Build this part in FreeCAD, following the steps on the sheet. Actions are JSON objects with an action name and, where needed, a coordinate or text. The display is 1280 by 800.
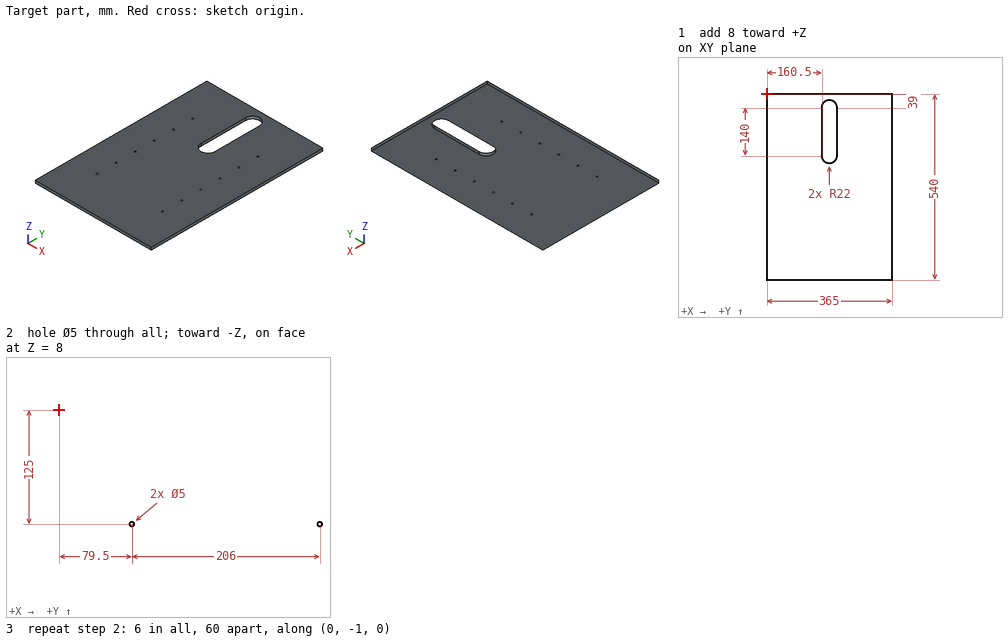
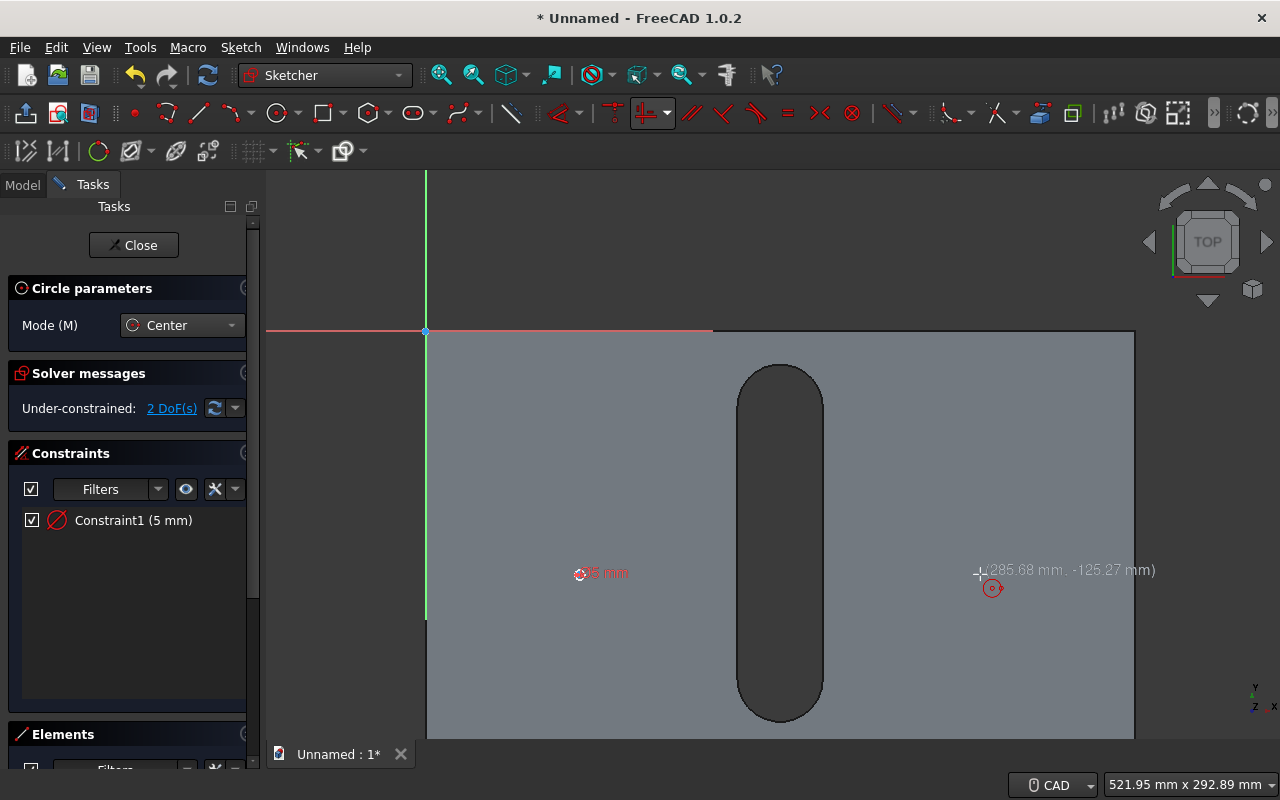
{"action": "left_click", "coordinate": [980, 574]}
{"action": "mouse_move", "coordinate": [984, 571]}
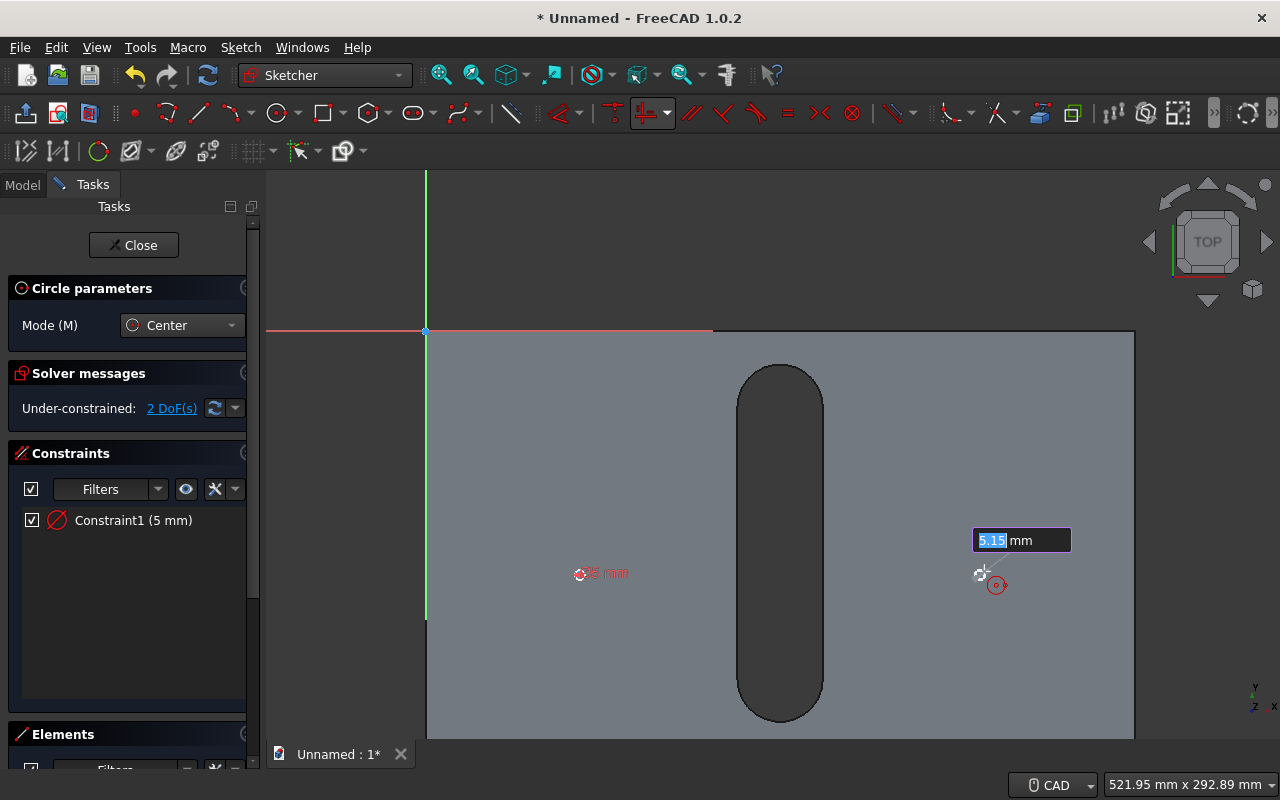
{"action": "type", "text": "5"}
{"action": "key", "text": "Return"}
{"action": "key", "text": "Escape"}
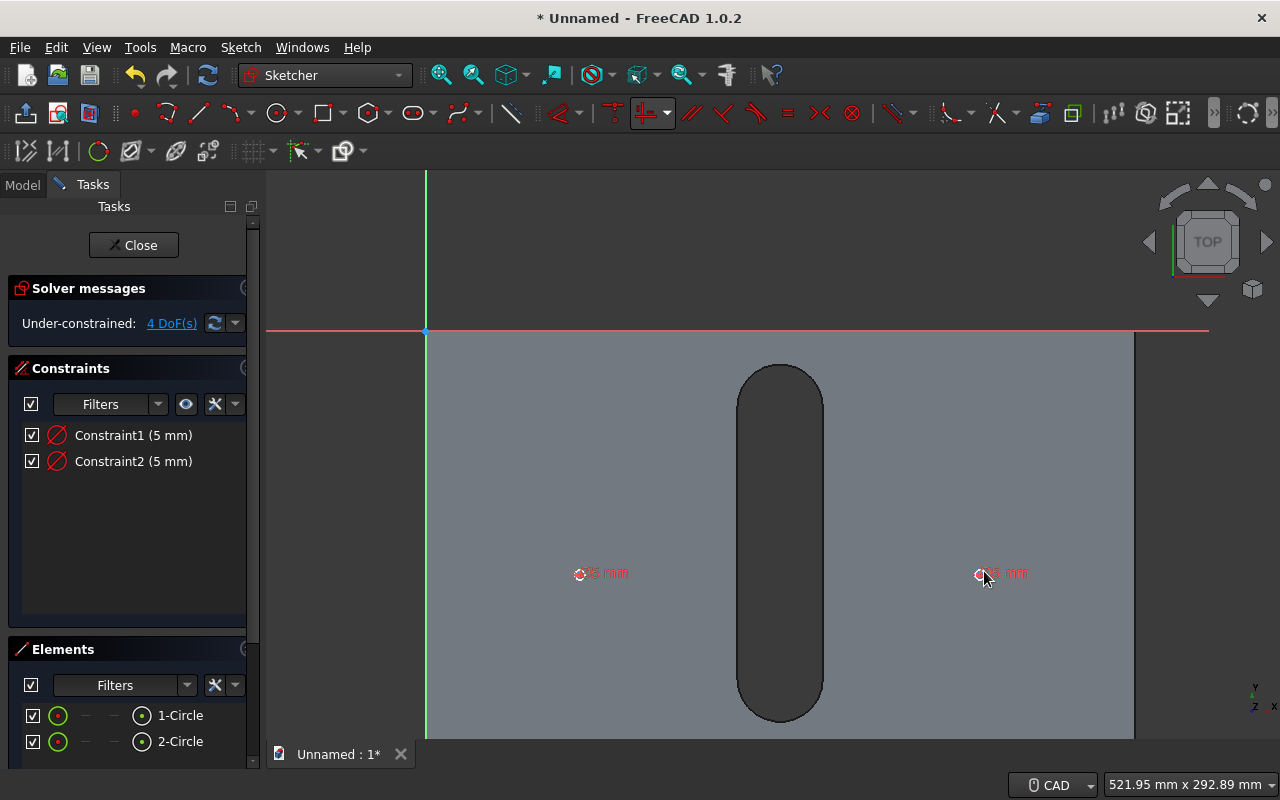
{"action": "left_click", "coordinate": [580, 575]}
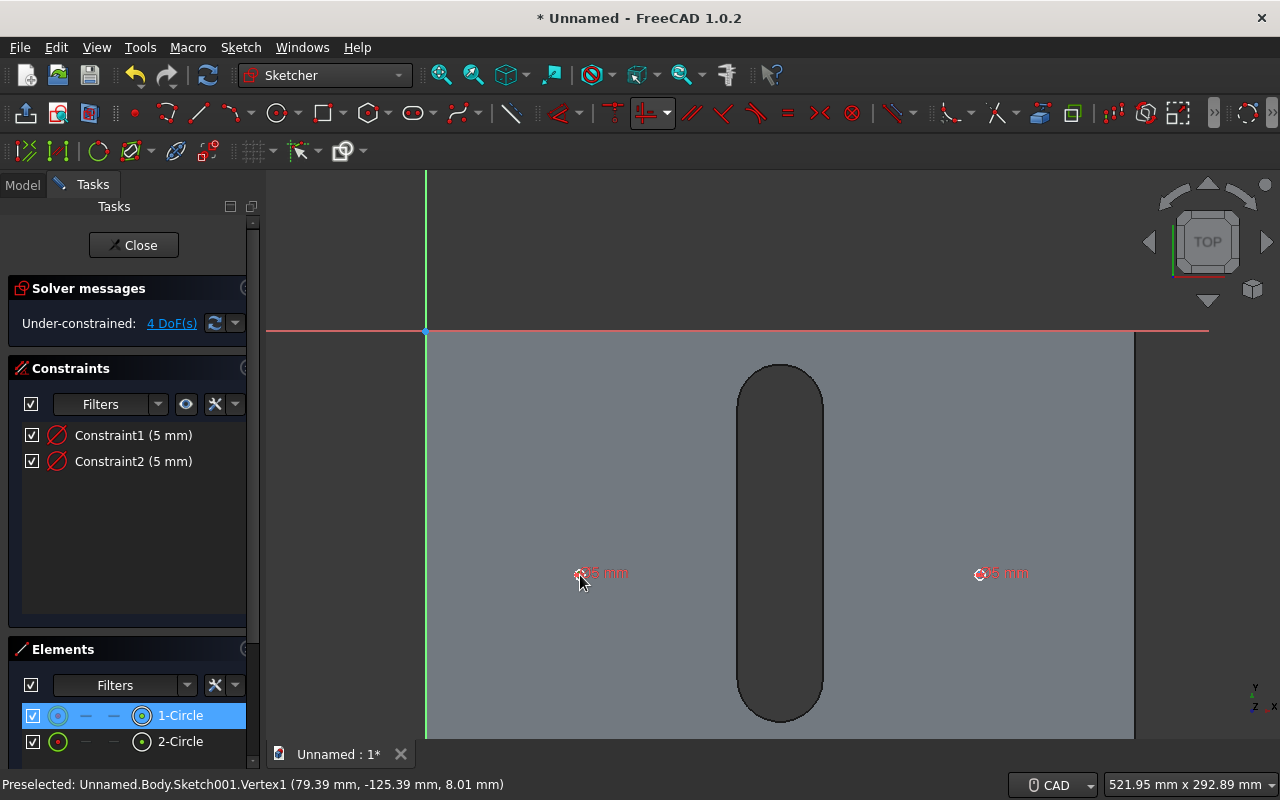
{"action": "left_click", "coordinate": [980, 575]}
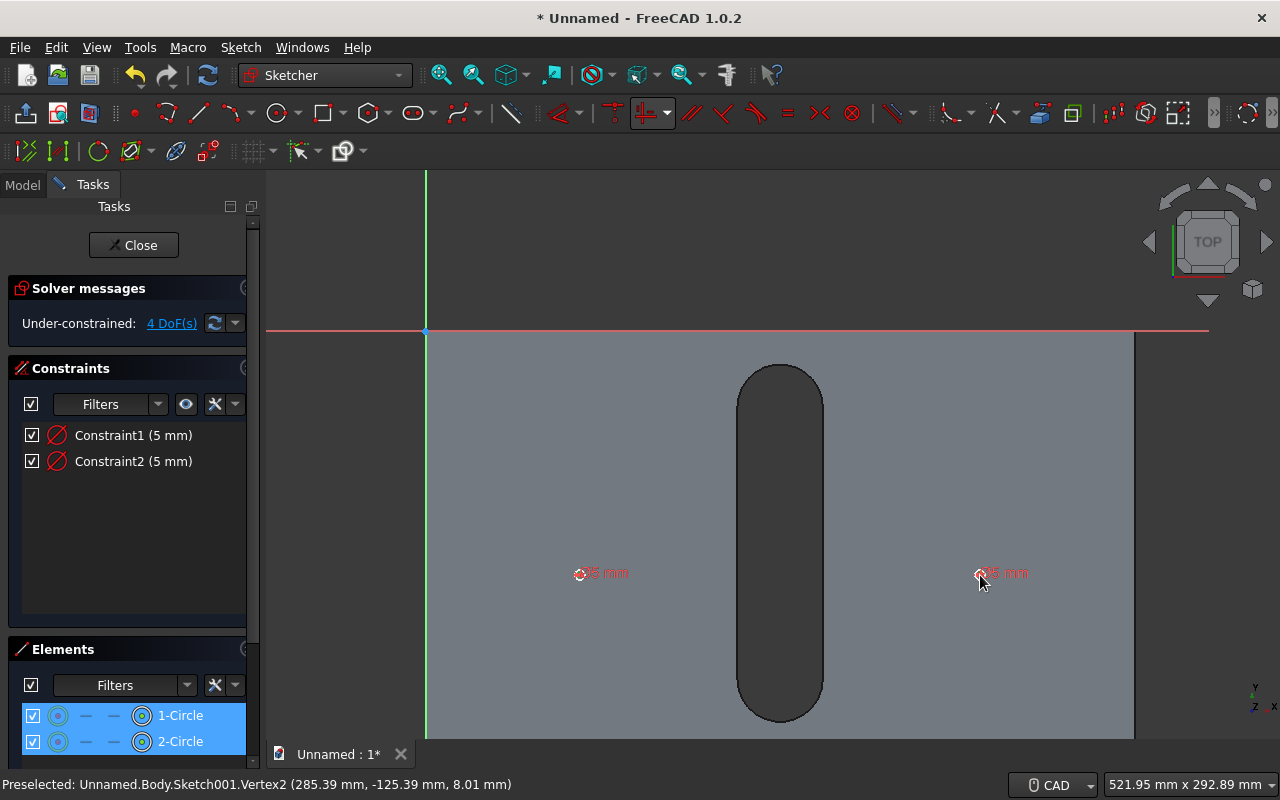
{"action": "key", "text": "h"}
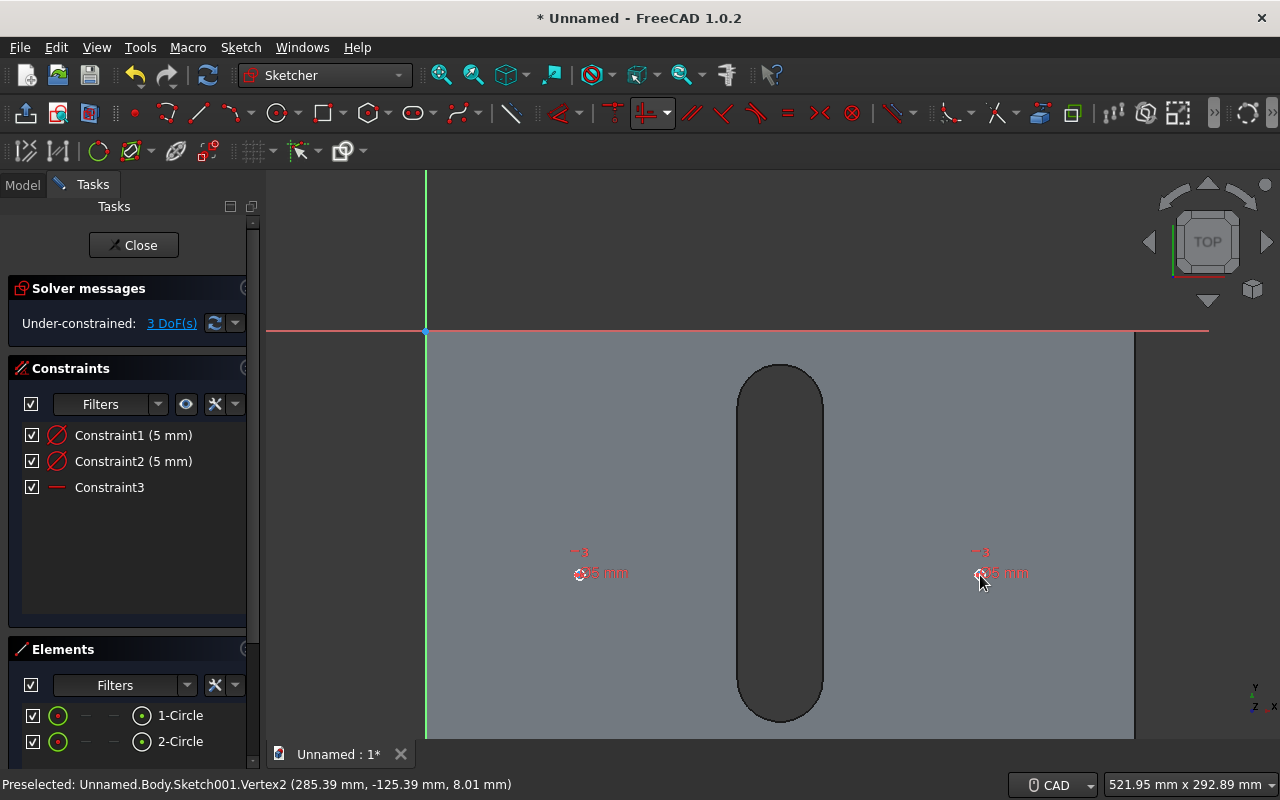
{"action": "left_click", "coordinate": [558, 114]}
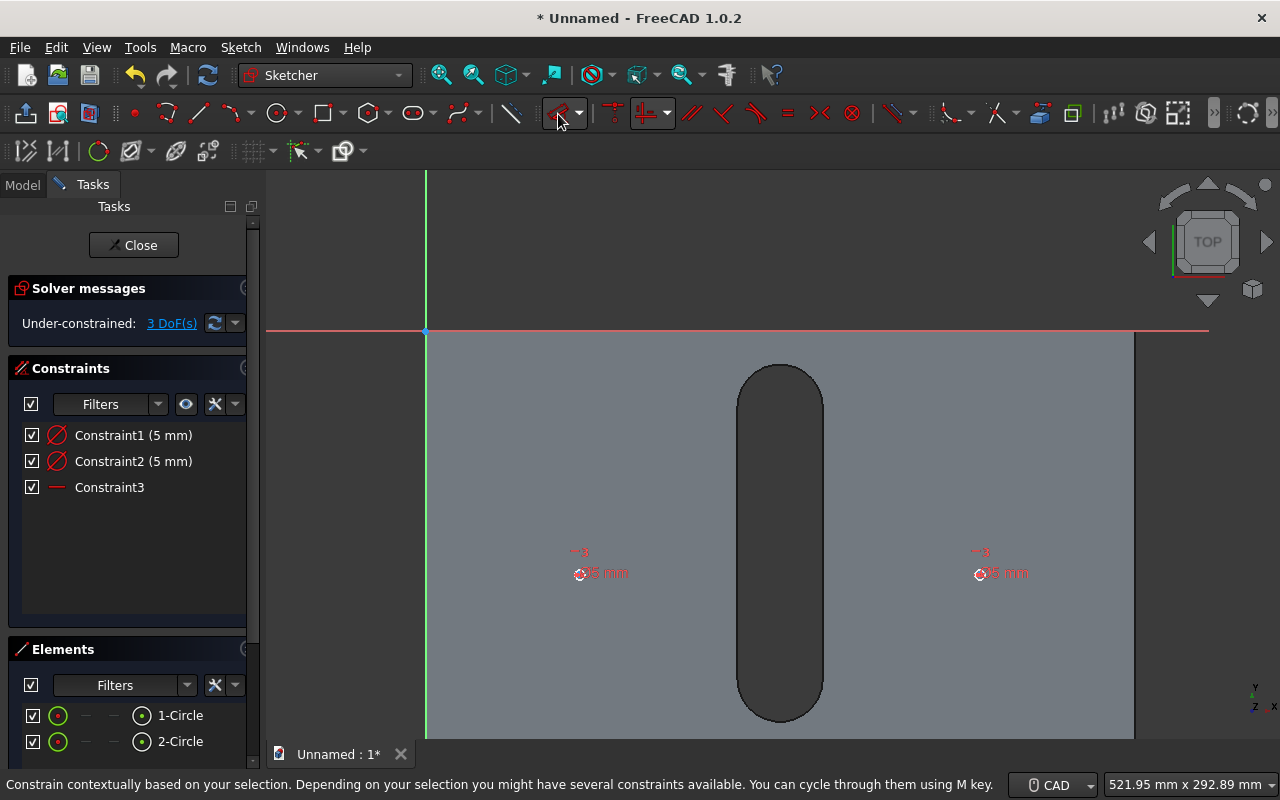
{"action": "left_click", "coordinate": [580, 575]}
{"action": "left_click", "coordinate": [392, 453]}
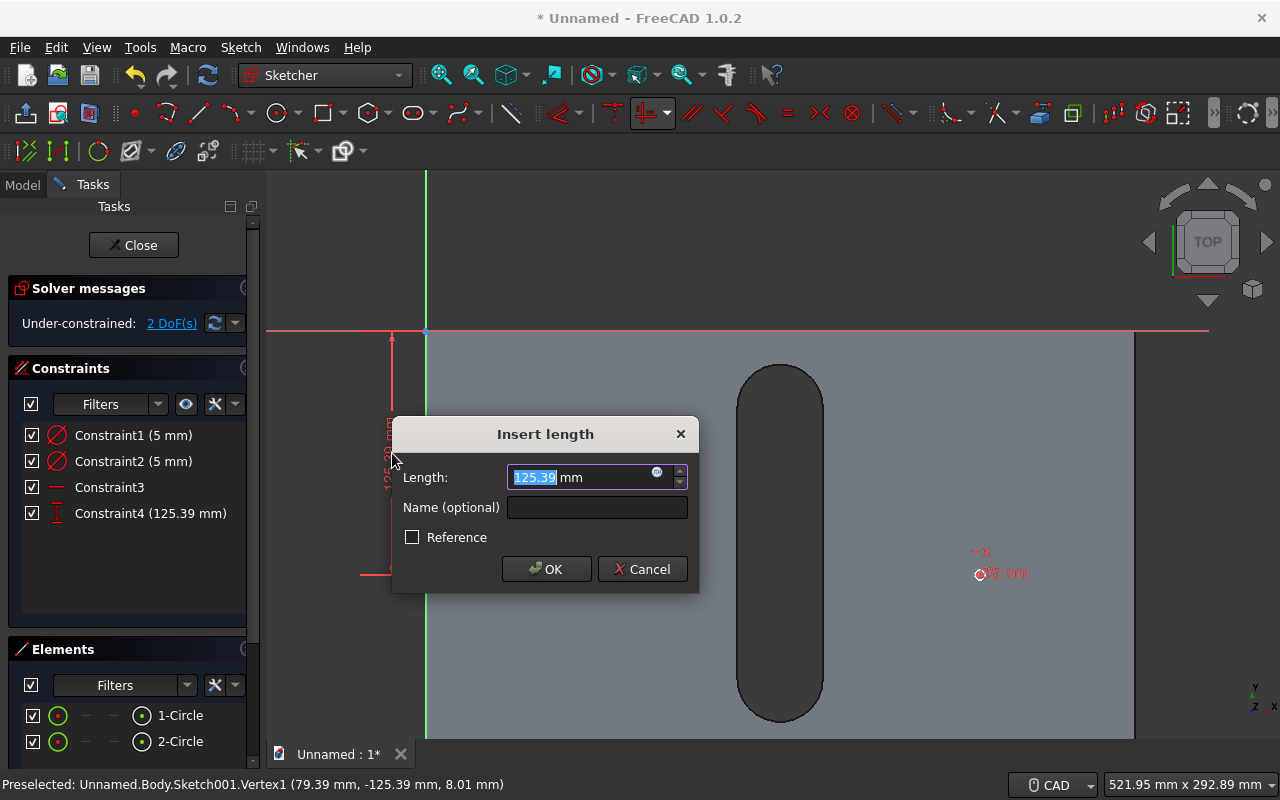
{"action": "type", "text": "125"}
{"action": "key", "text": "Return"}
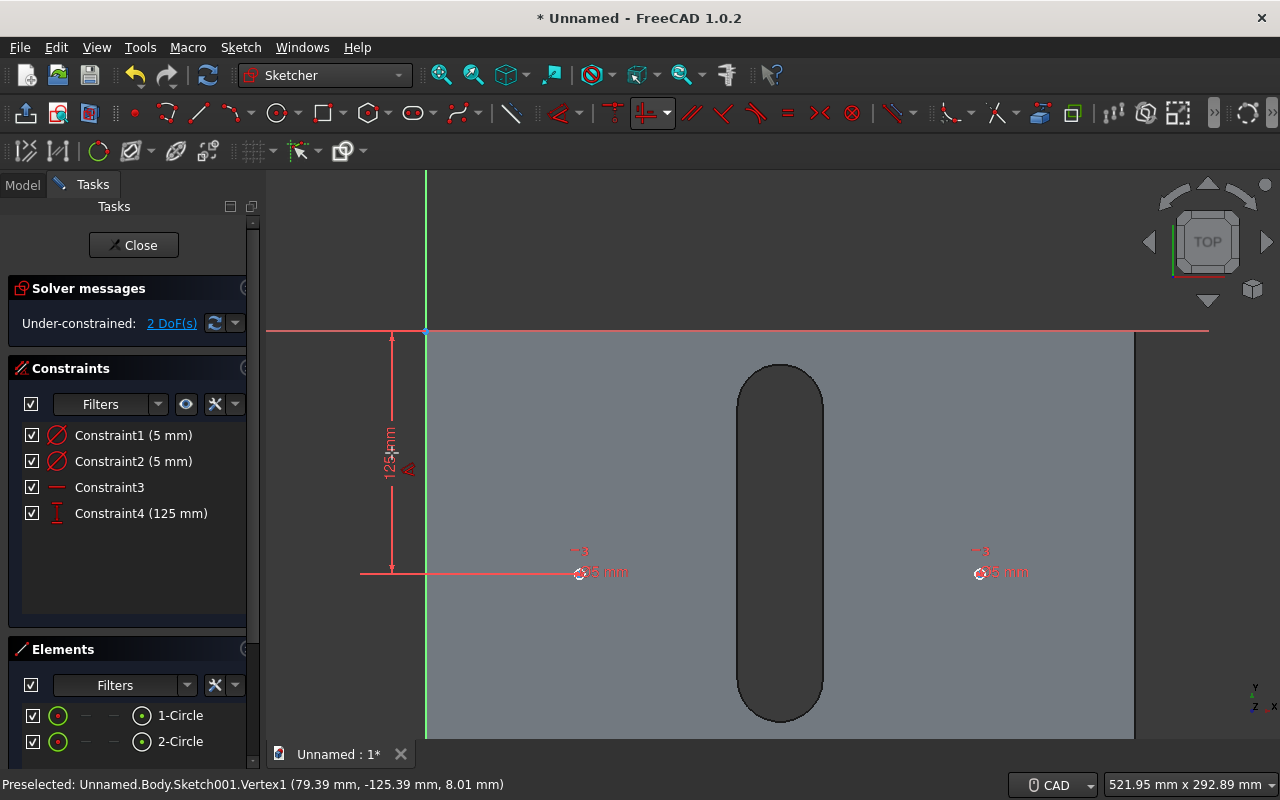
{"action": "left_click", "coordinate": [580, 574]}
{"action": "left_click", "coordinate": [503, 297]}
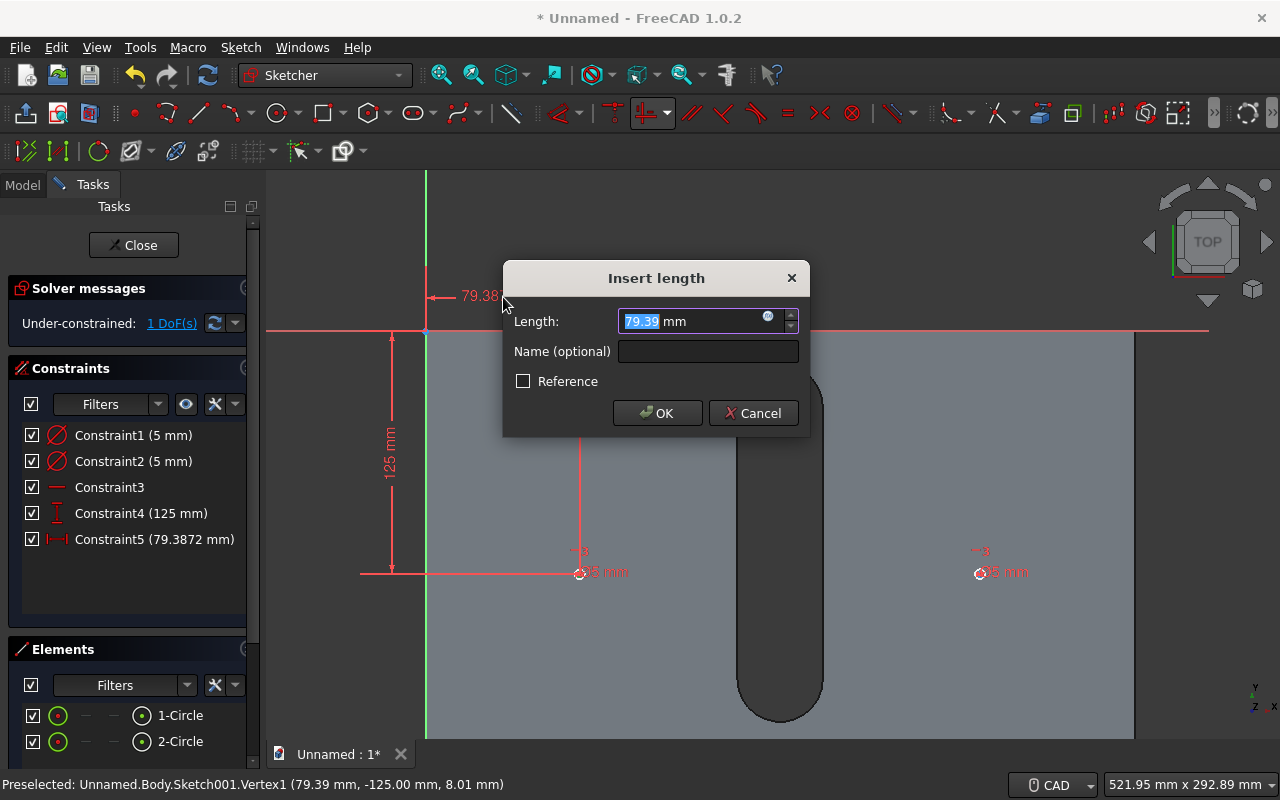
{"action": "type", "text": "79.5"}
{"action": "key", "text": "Return"}